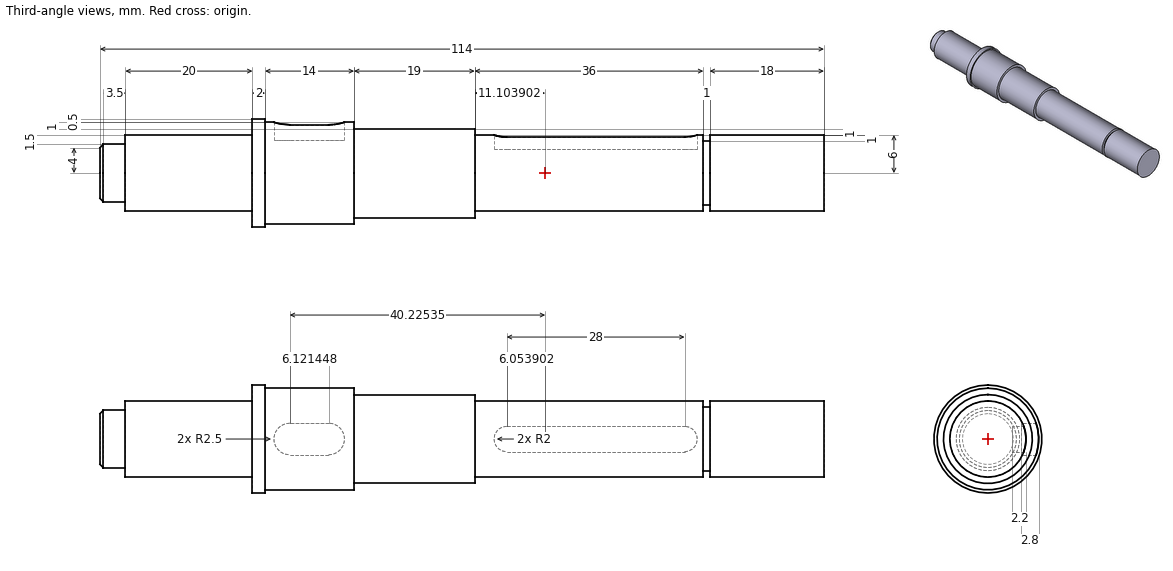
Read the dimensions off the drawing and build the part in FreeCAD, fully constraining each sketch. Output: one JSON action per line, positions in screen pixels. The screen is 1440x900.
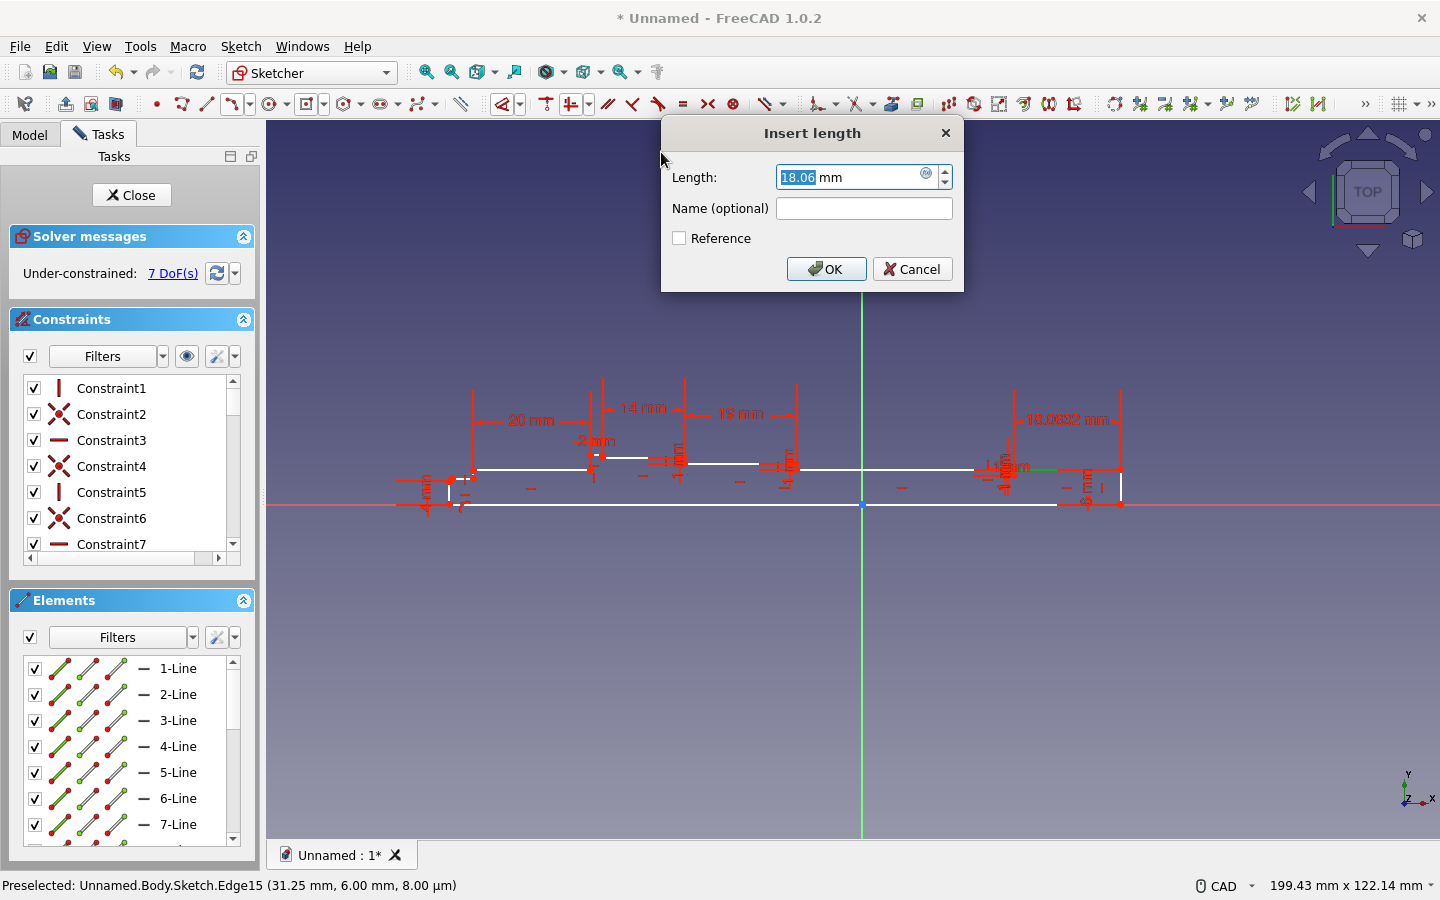
{"action": "type", "text": "18"}
{"action": "key", "text": "Return"}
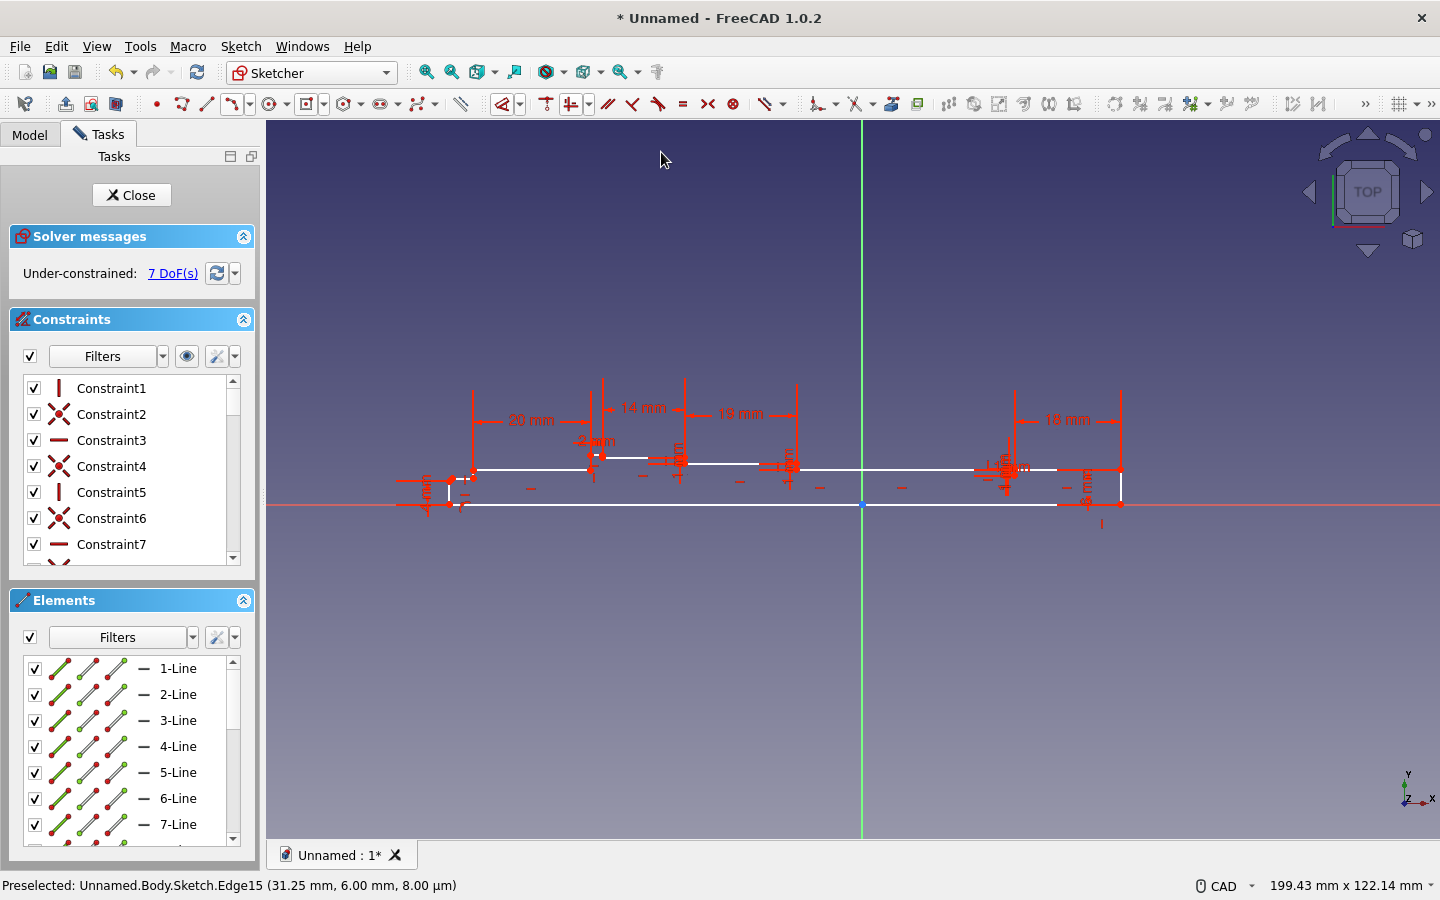
{"action": "left_click", "coordinate": [945, 470]}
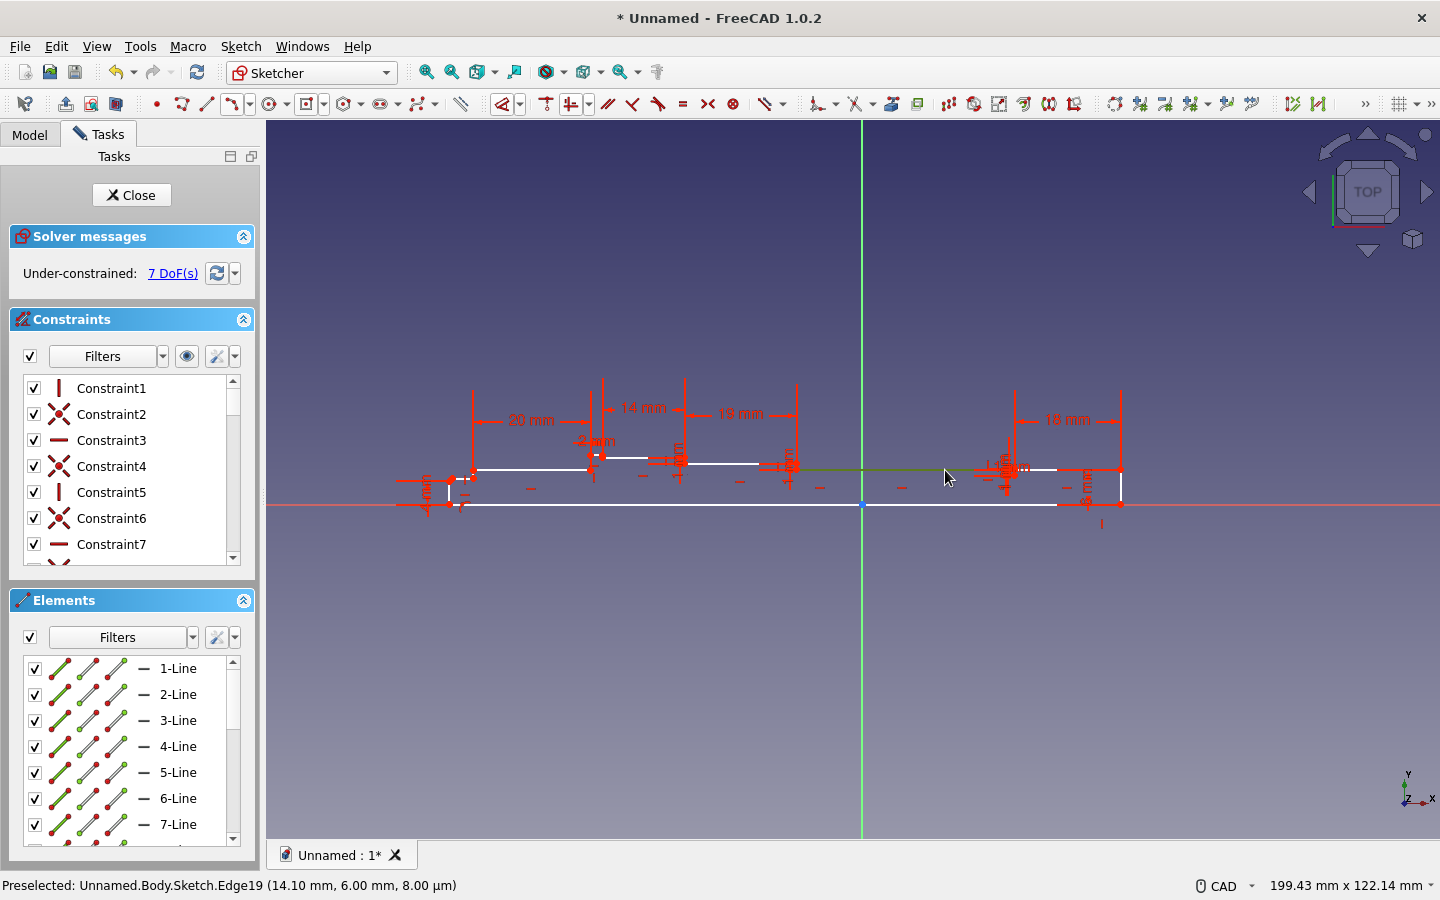
{"action": "key", "text": "l"}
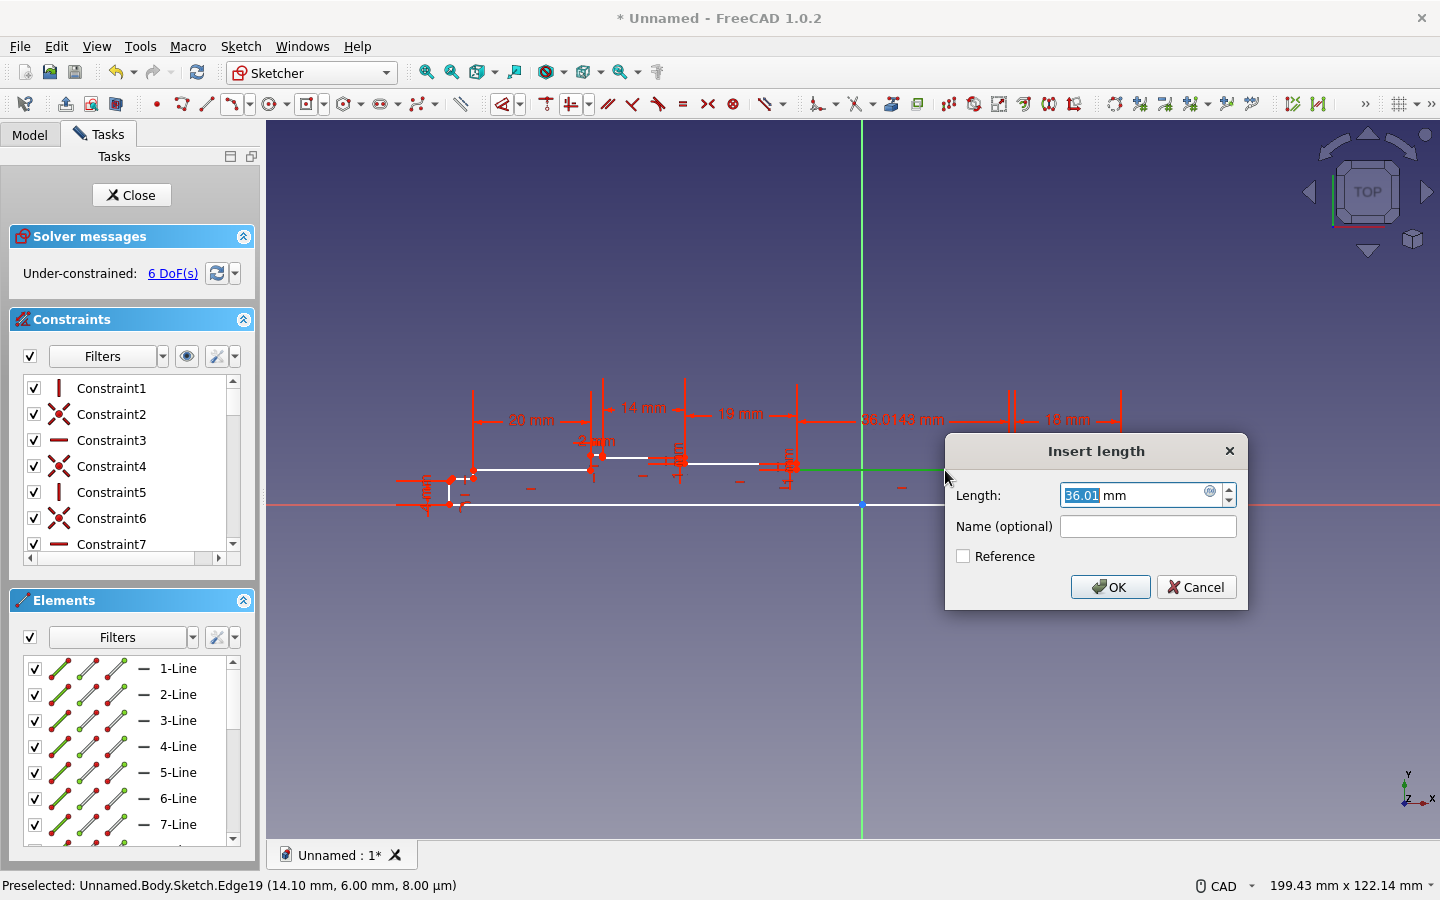
{"action": "type", "text": "36"}
{"action": "key", "text": "Return"}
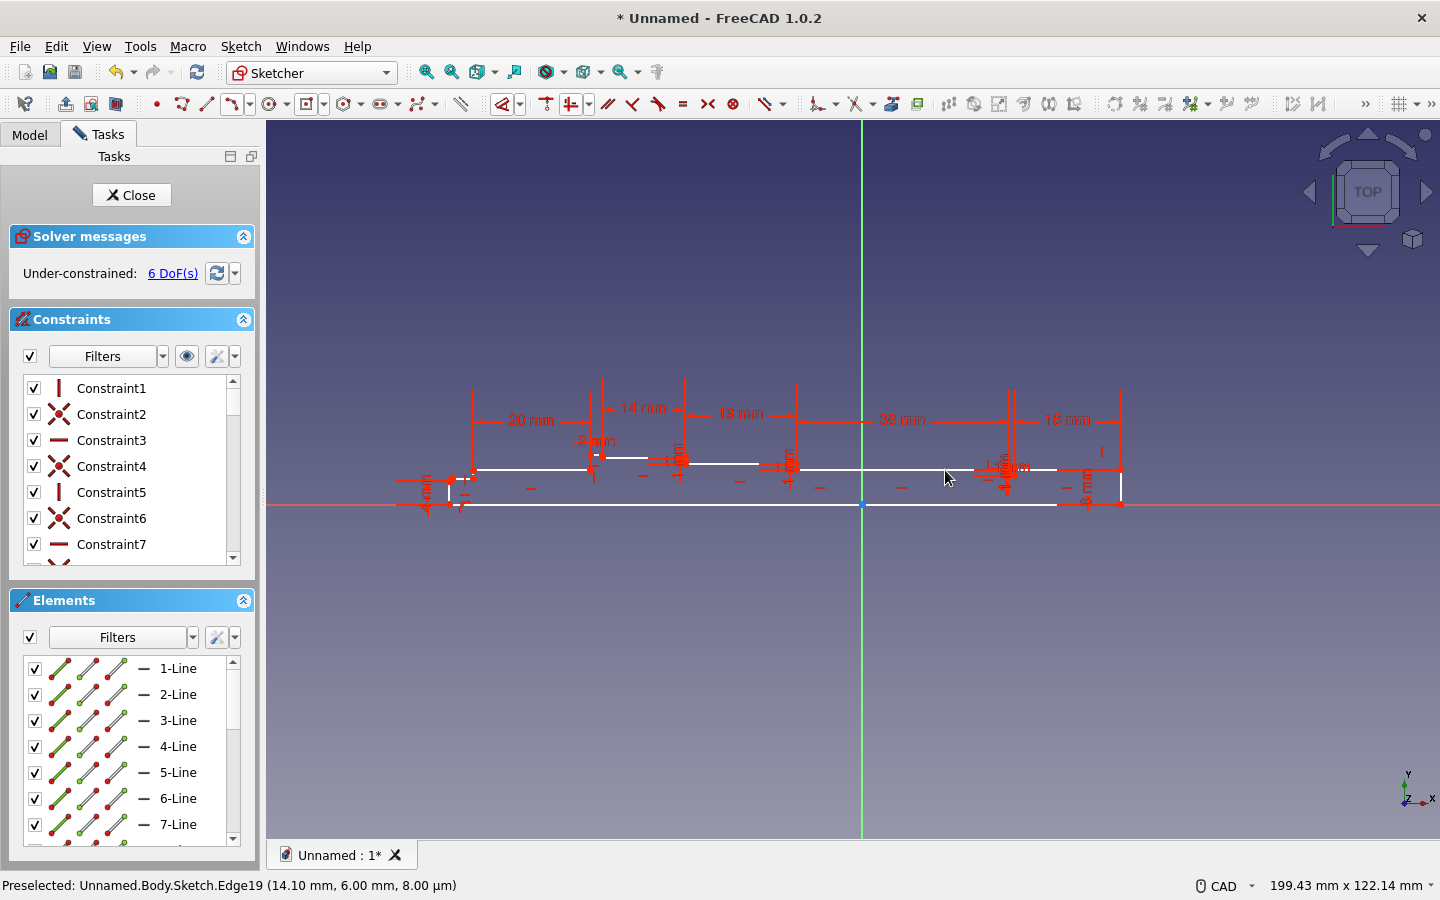
{"action": "left_click", "coordinate": [591, 470]}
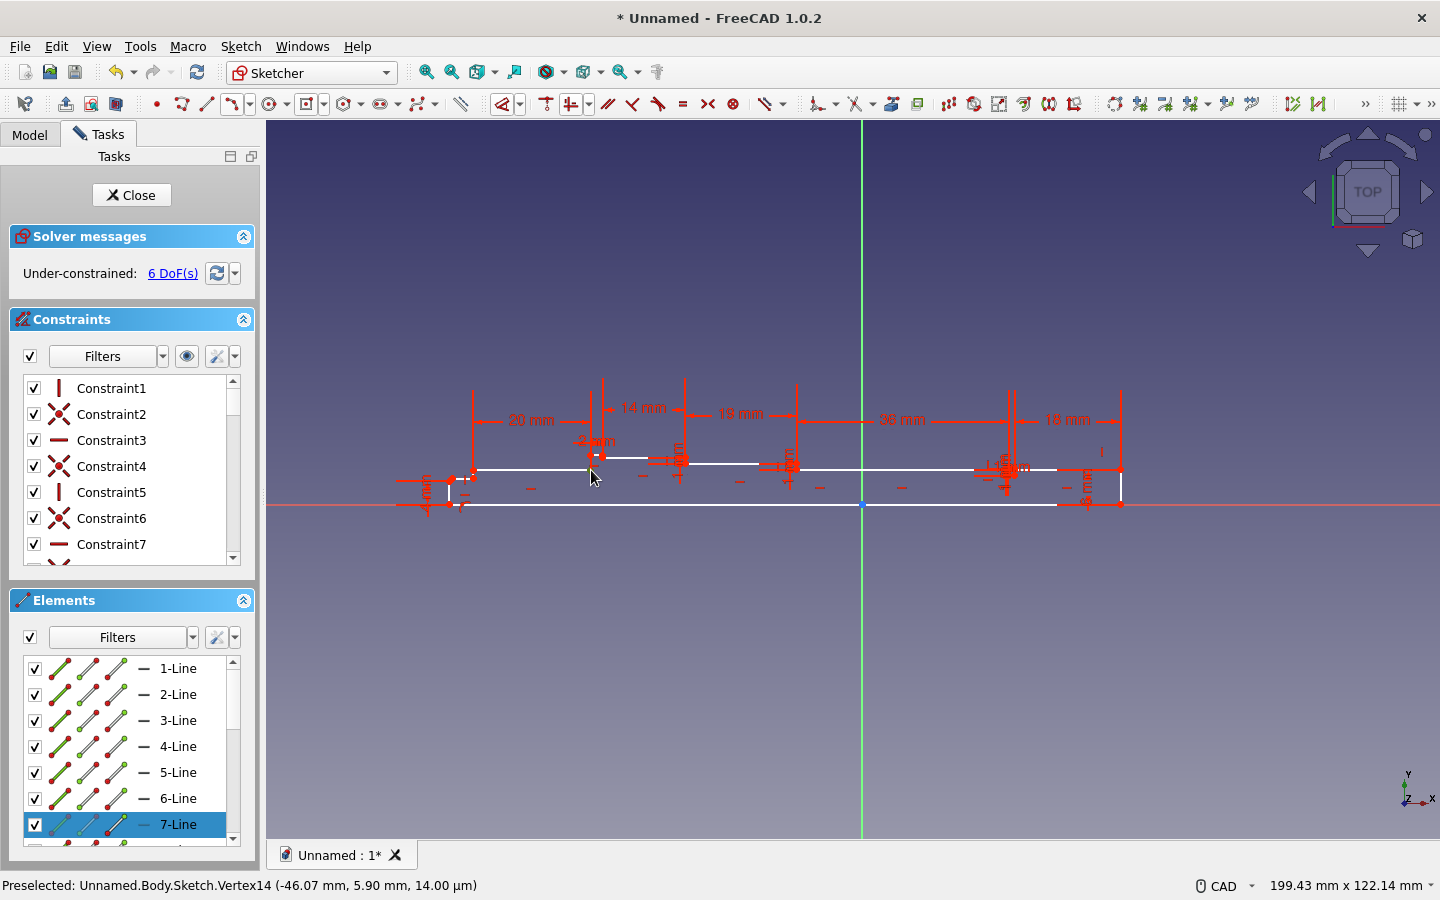
{"action": "key", "text": "i"}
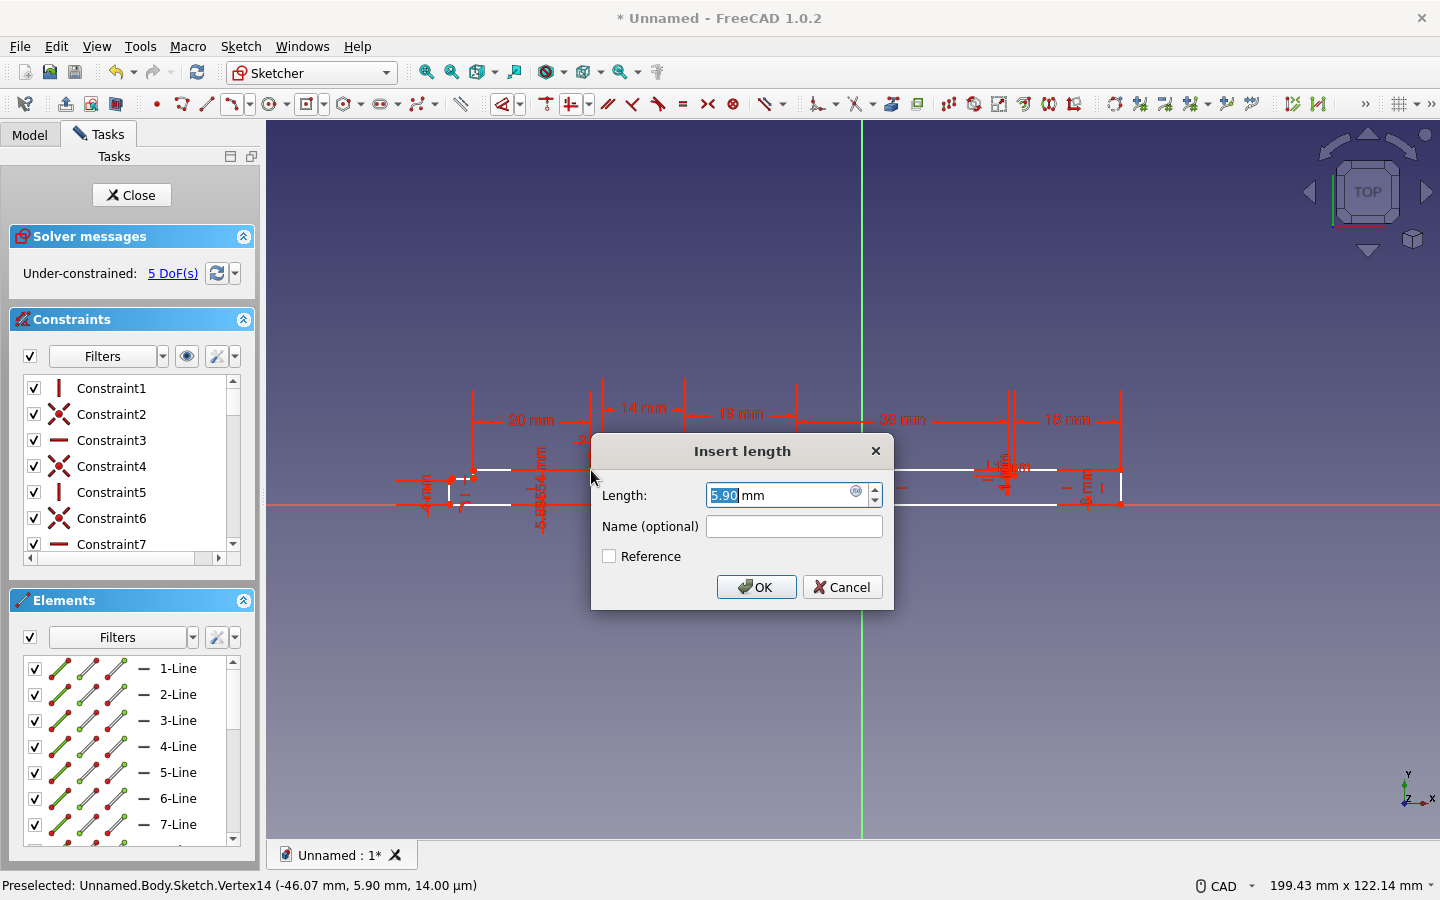
{"action": "type", "text": "6"}
{"action": "key", "text": "Return"}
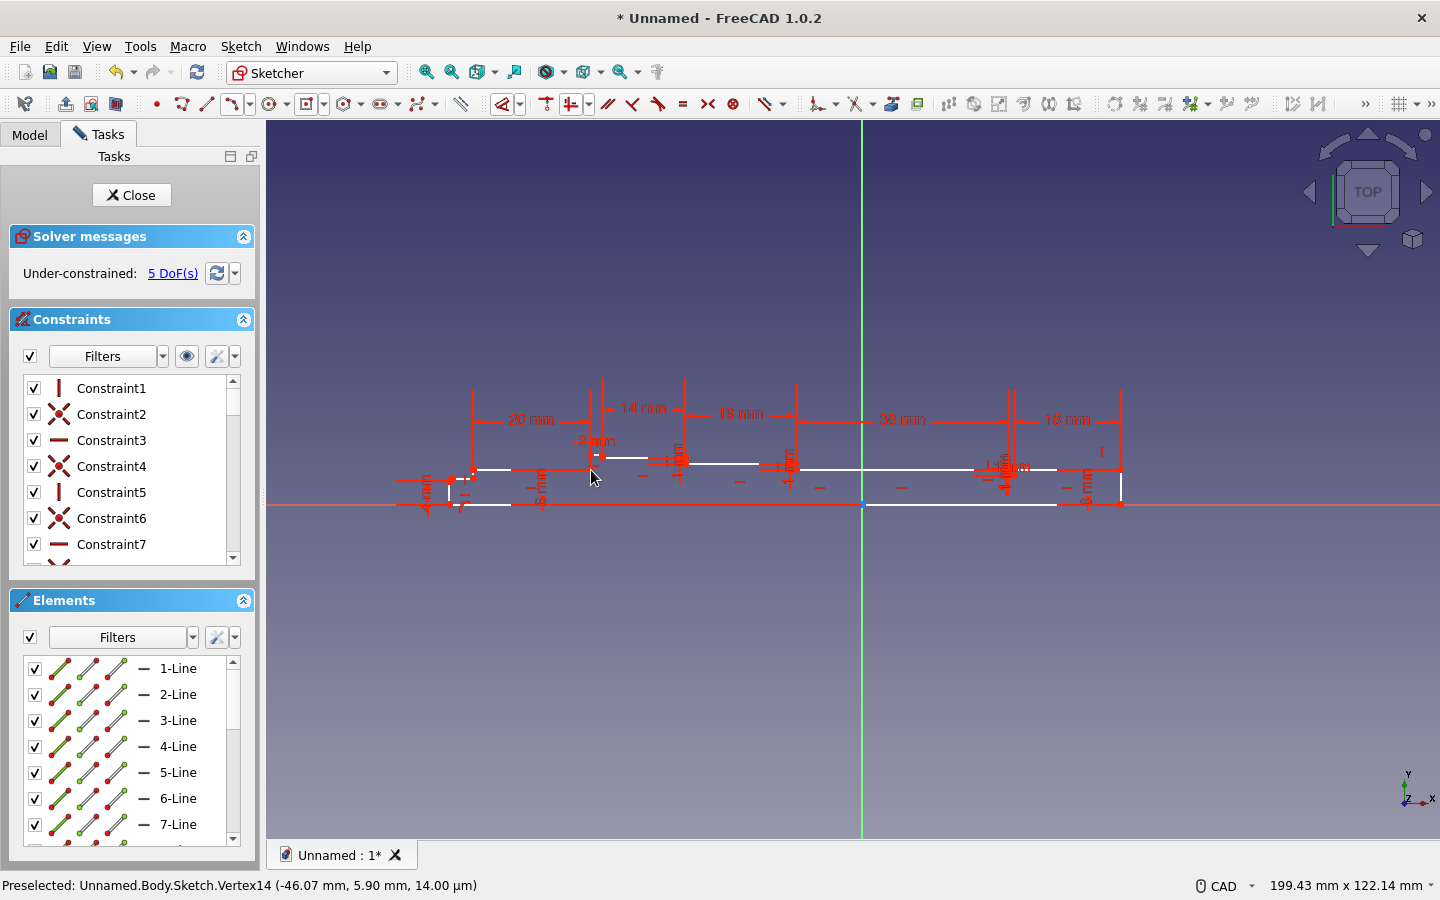
{"action": "scroll", "coordinate": [603, 456], "scroll_direction": "up", "scroll_amount": 14}